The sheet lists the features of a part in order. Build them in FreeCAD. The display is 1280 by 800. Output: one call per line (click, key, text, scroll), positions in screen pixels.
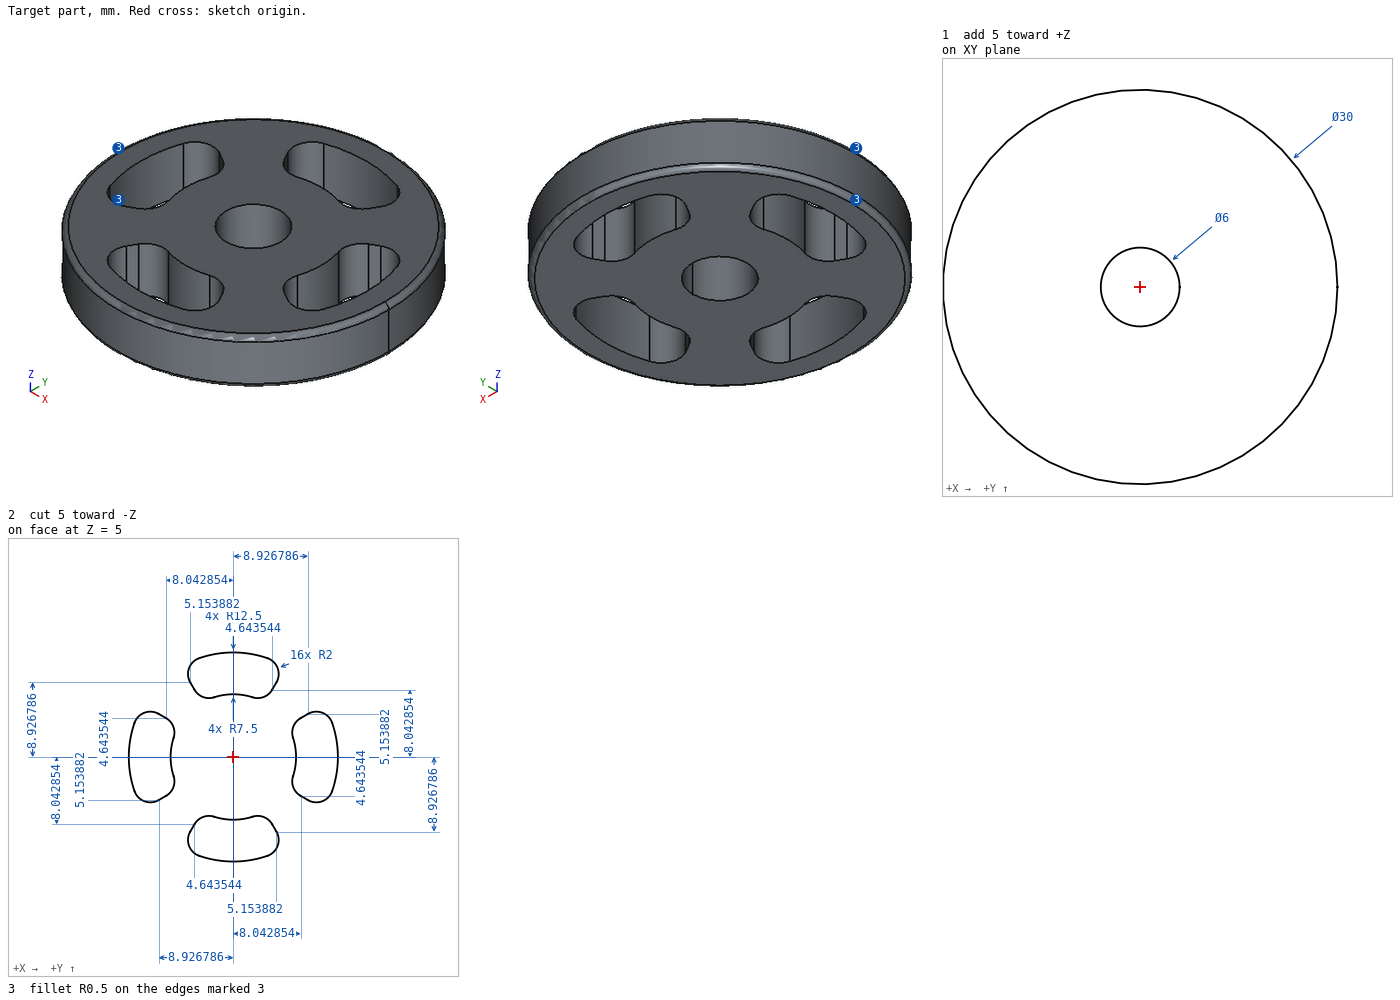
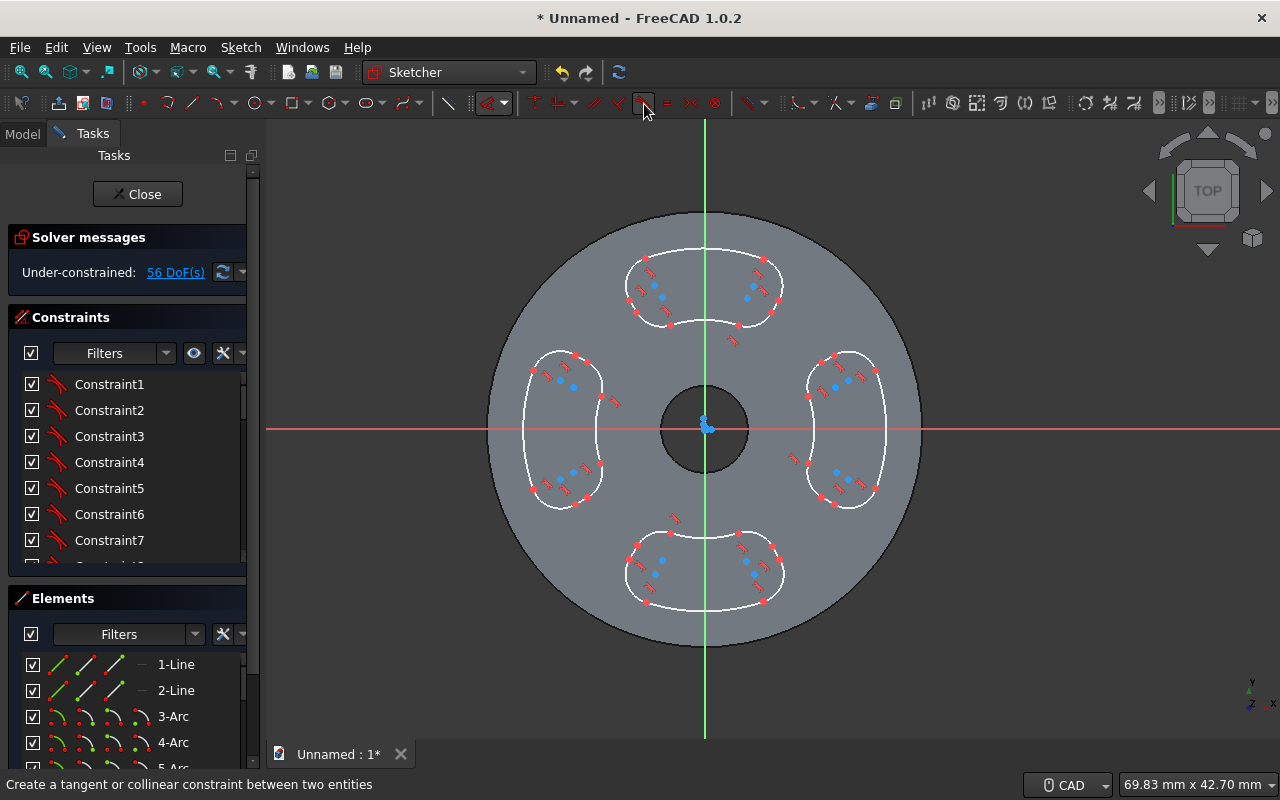
click(719, 321)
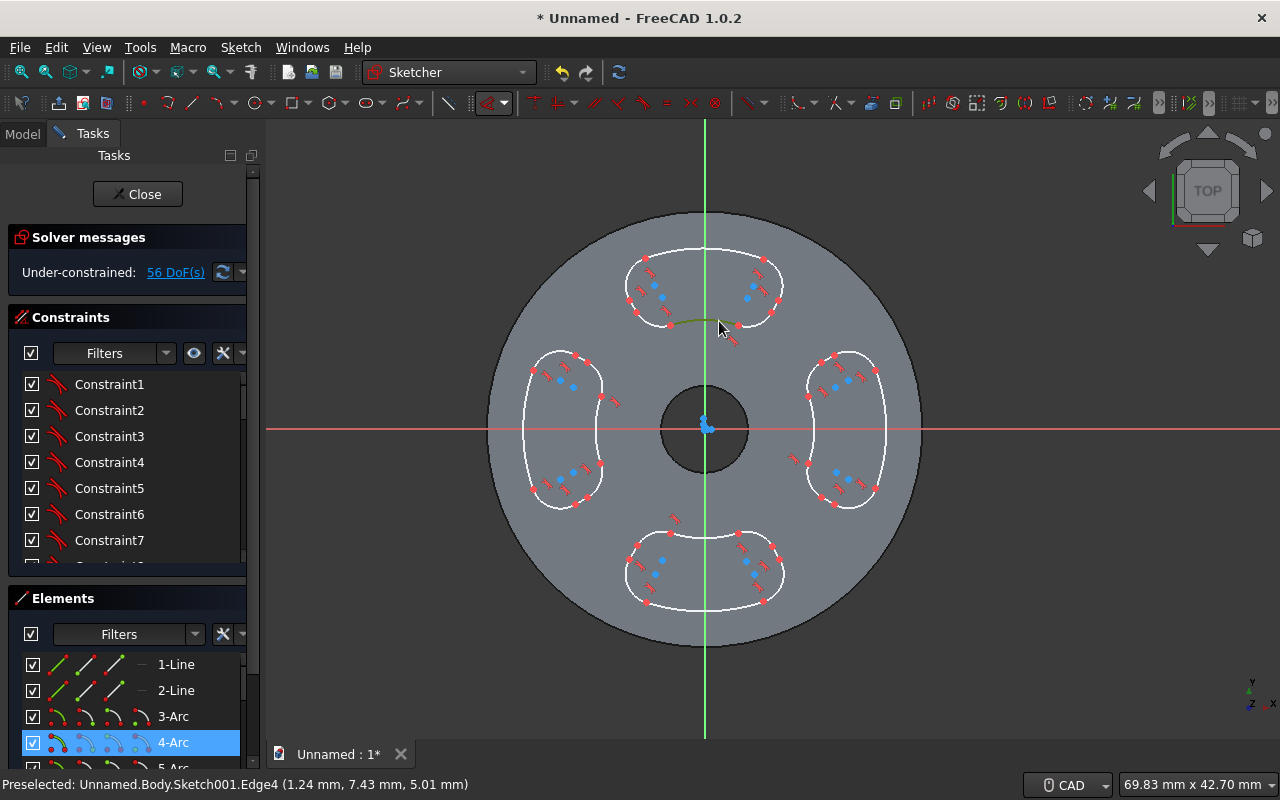
click(729, 250)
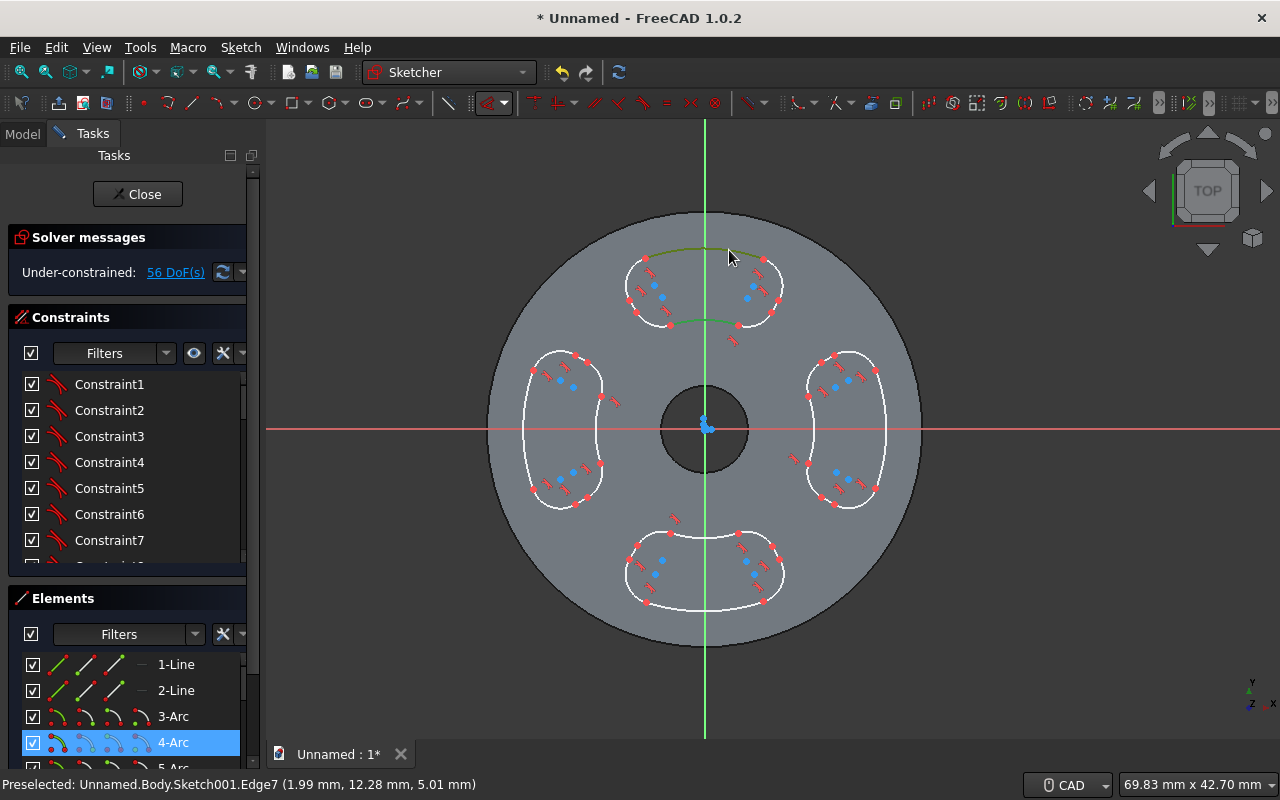
click(534, 104)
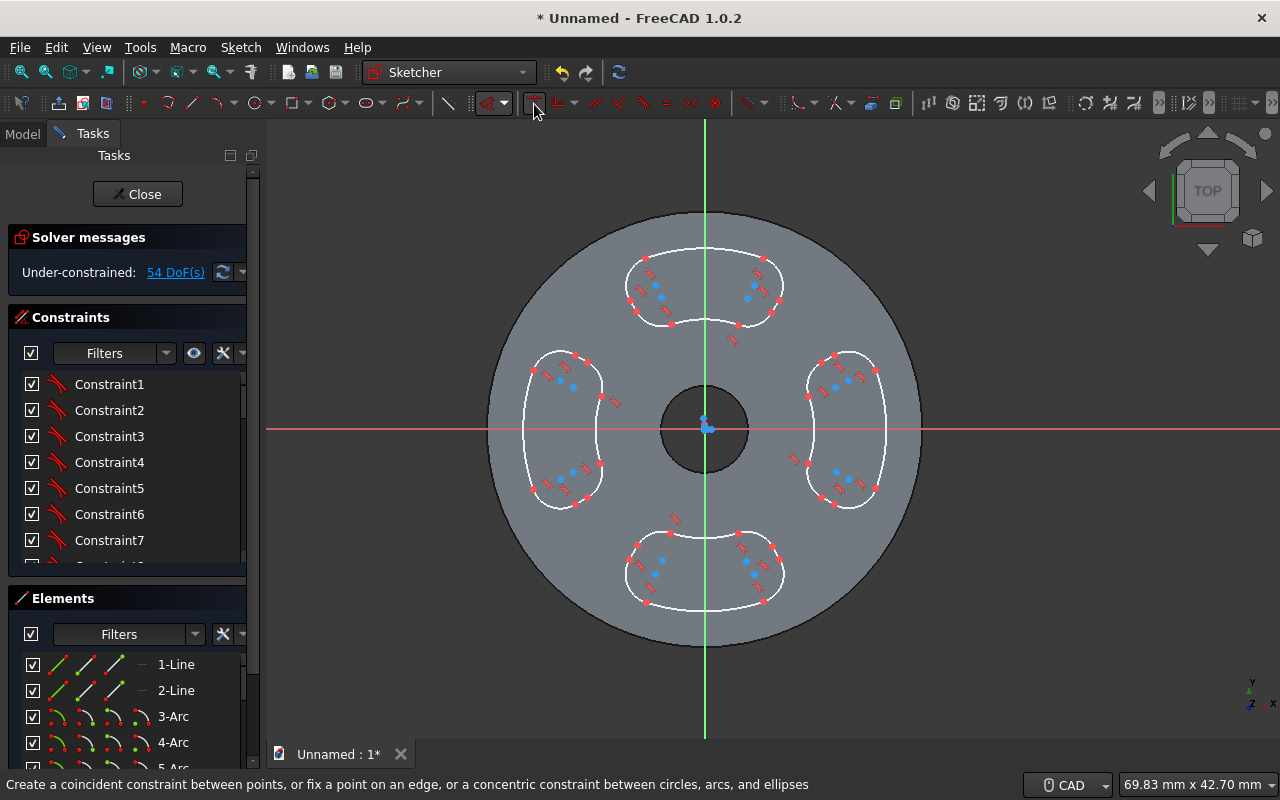
click(719, 320)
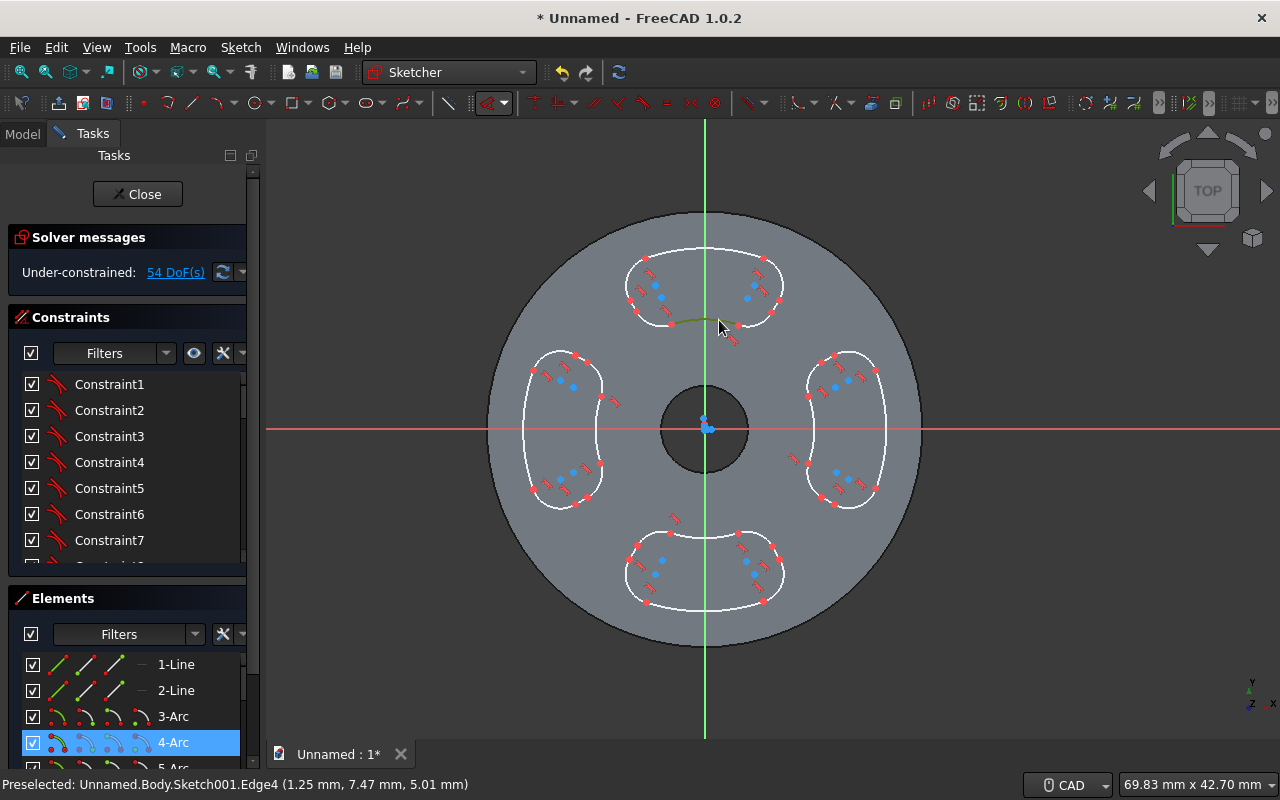
click(813, 443)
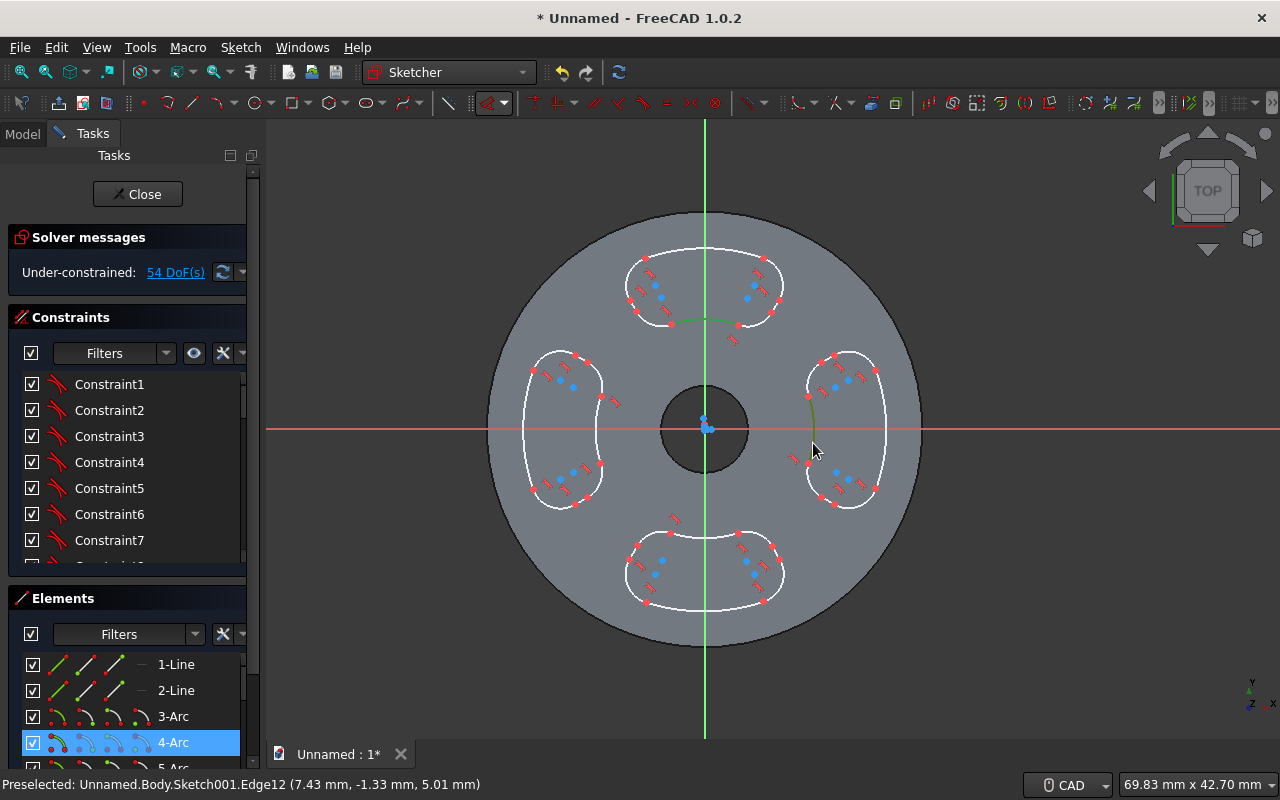
click(534, 104)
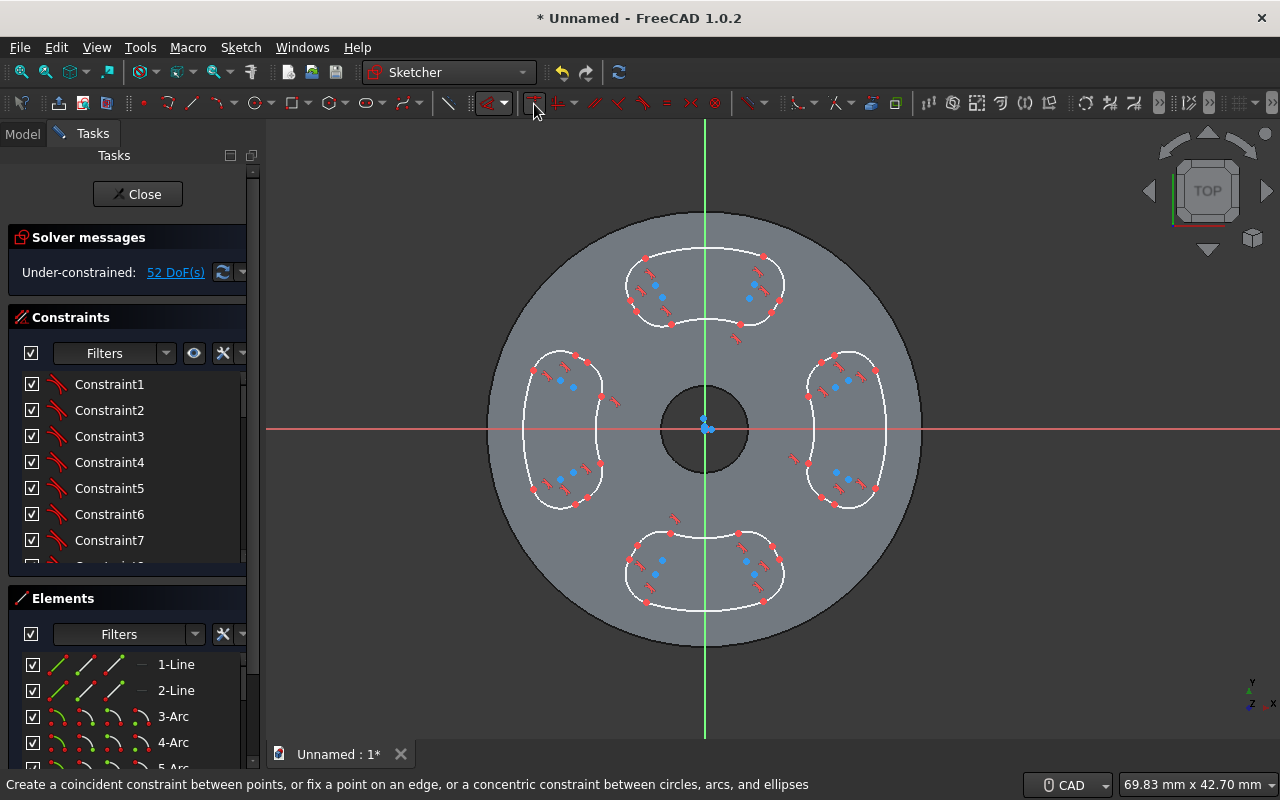
click(720, 320)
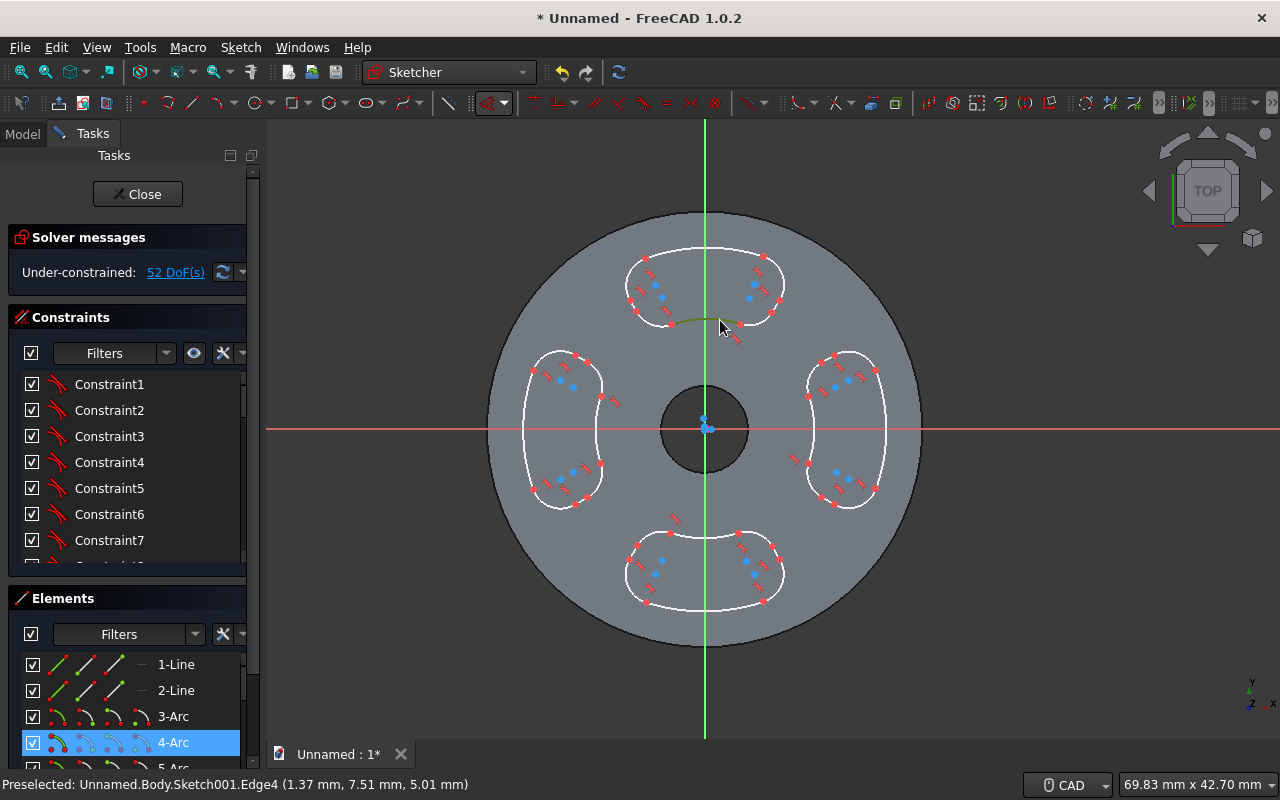
click(885, 454)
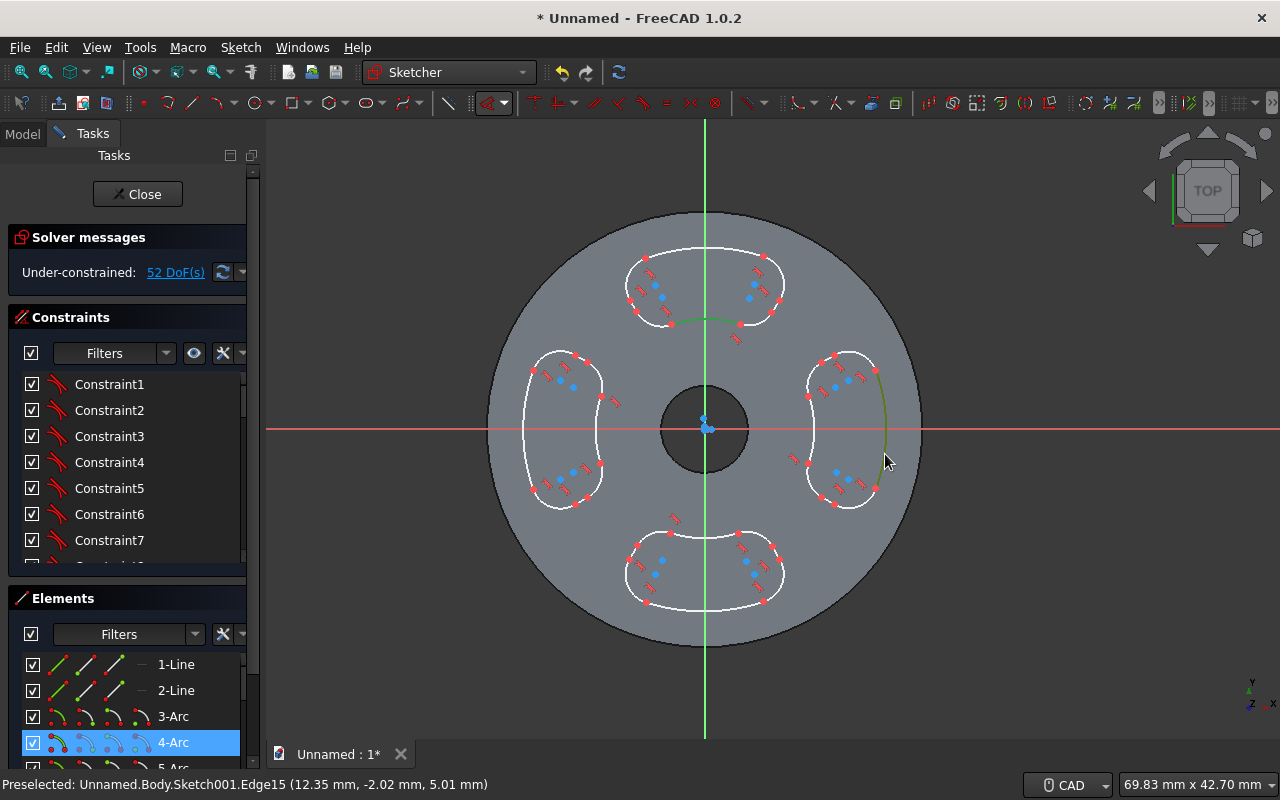
click(534, 104)